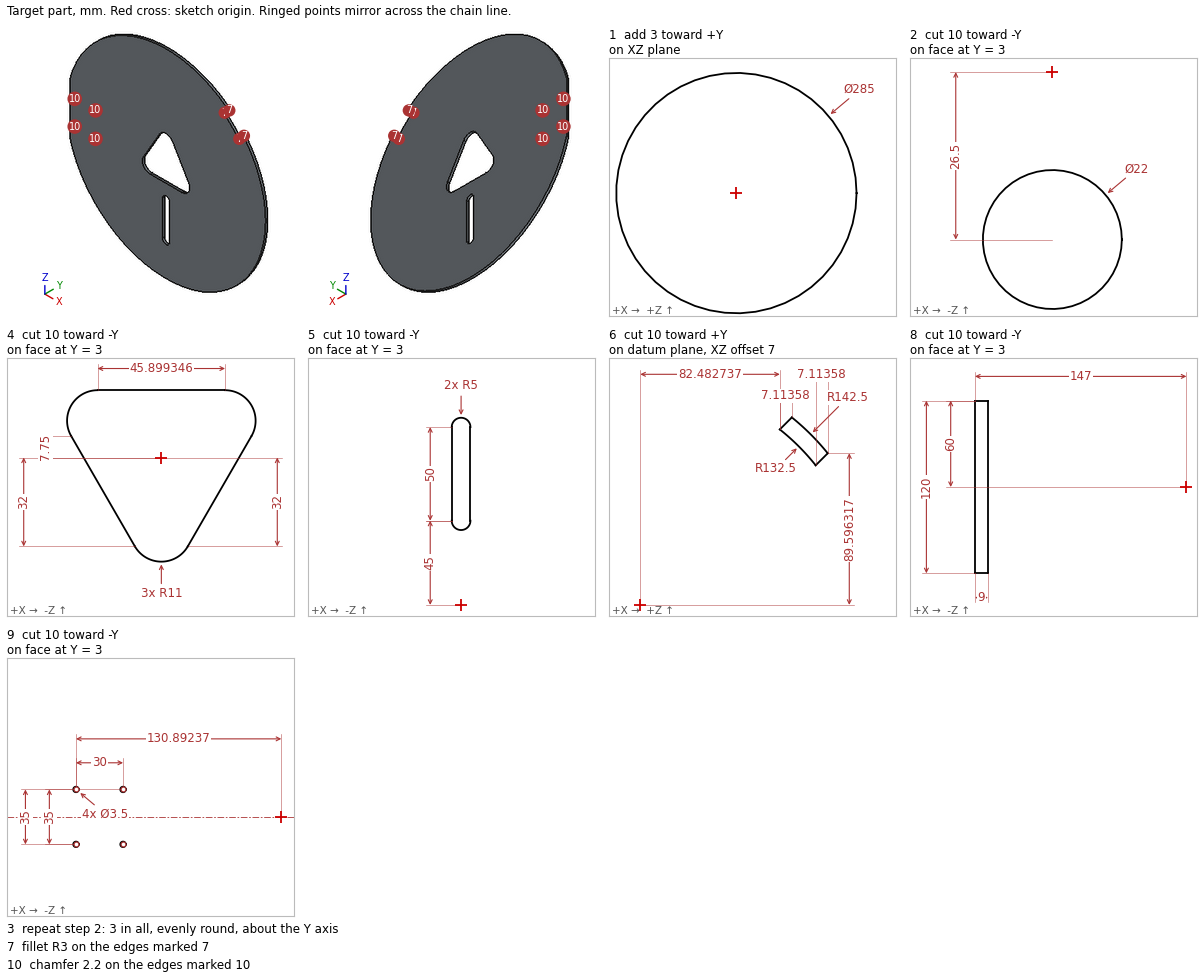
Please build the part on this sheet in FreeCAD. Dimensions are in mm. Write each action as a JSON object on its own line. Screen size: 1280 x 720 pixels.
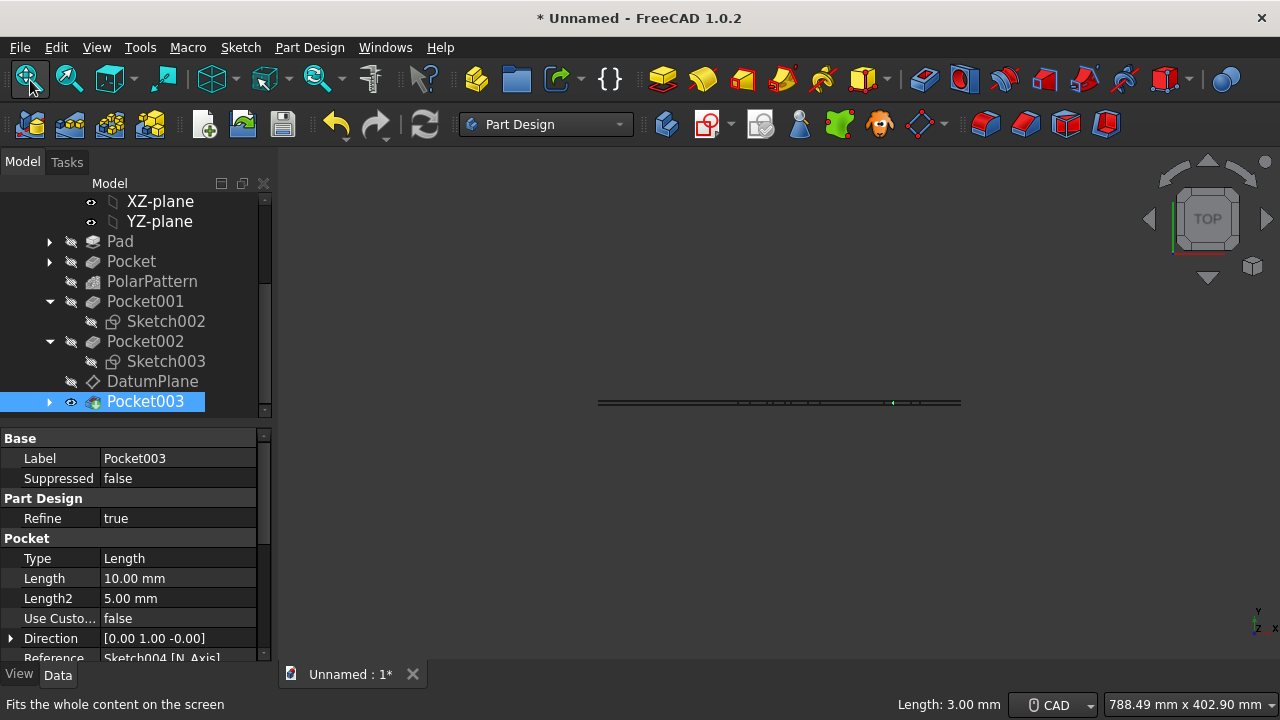
{"action": "scroll", "coordinate": [884, 402], "scroll_direction": "up", "scroll_amount": 12}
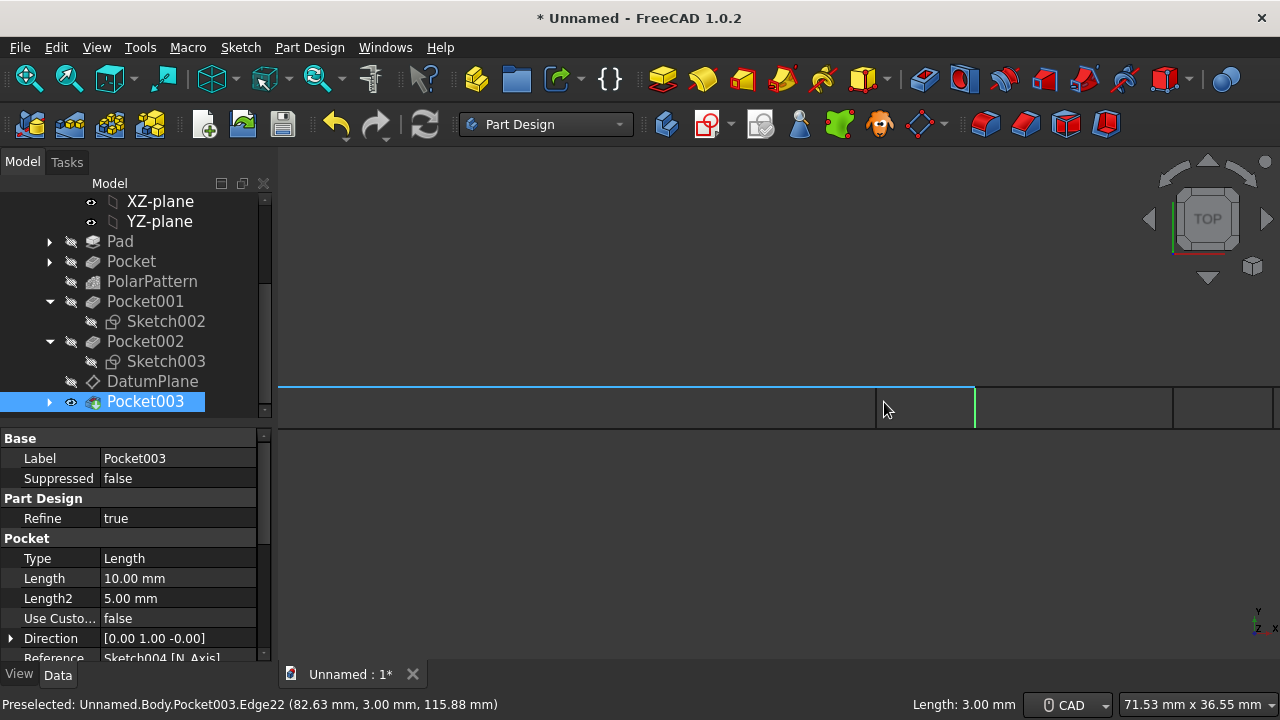
{"action": "left_click", "coordinate": [876, 407], "text": "ctrl"}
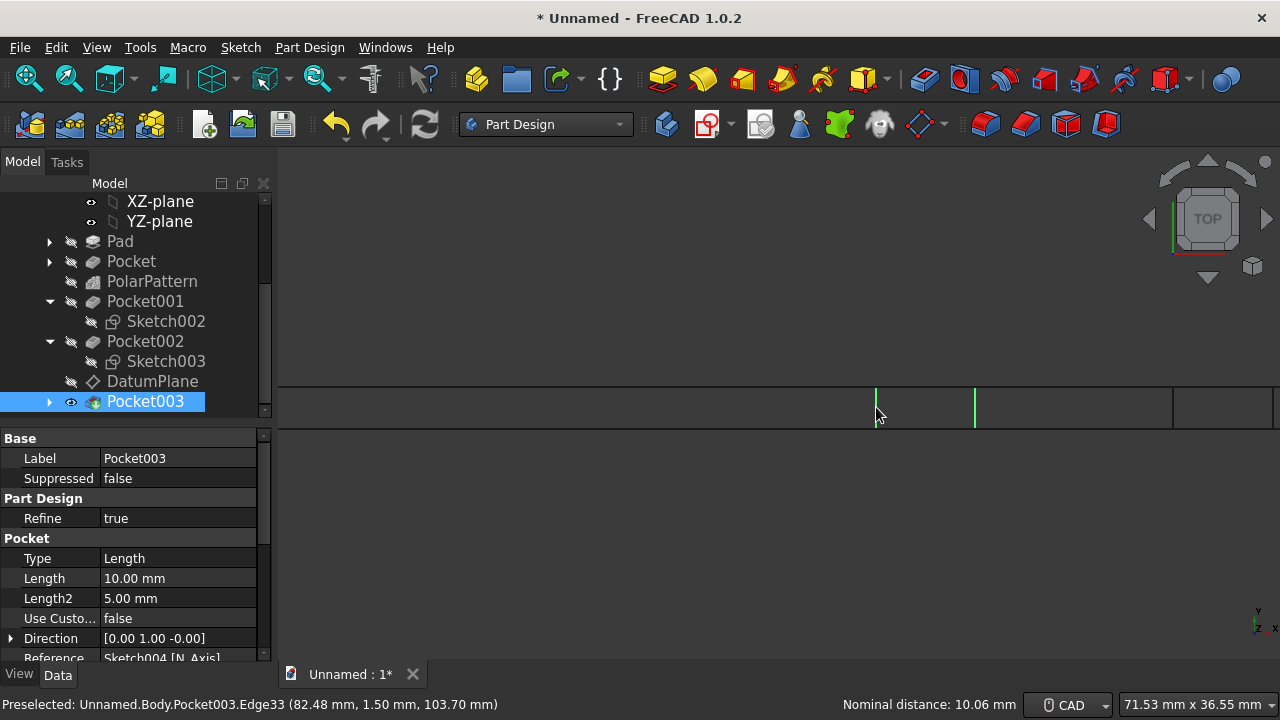
{"action": "left_click", "coordinate": [1173, 407], "text": "ctrl"}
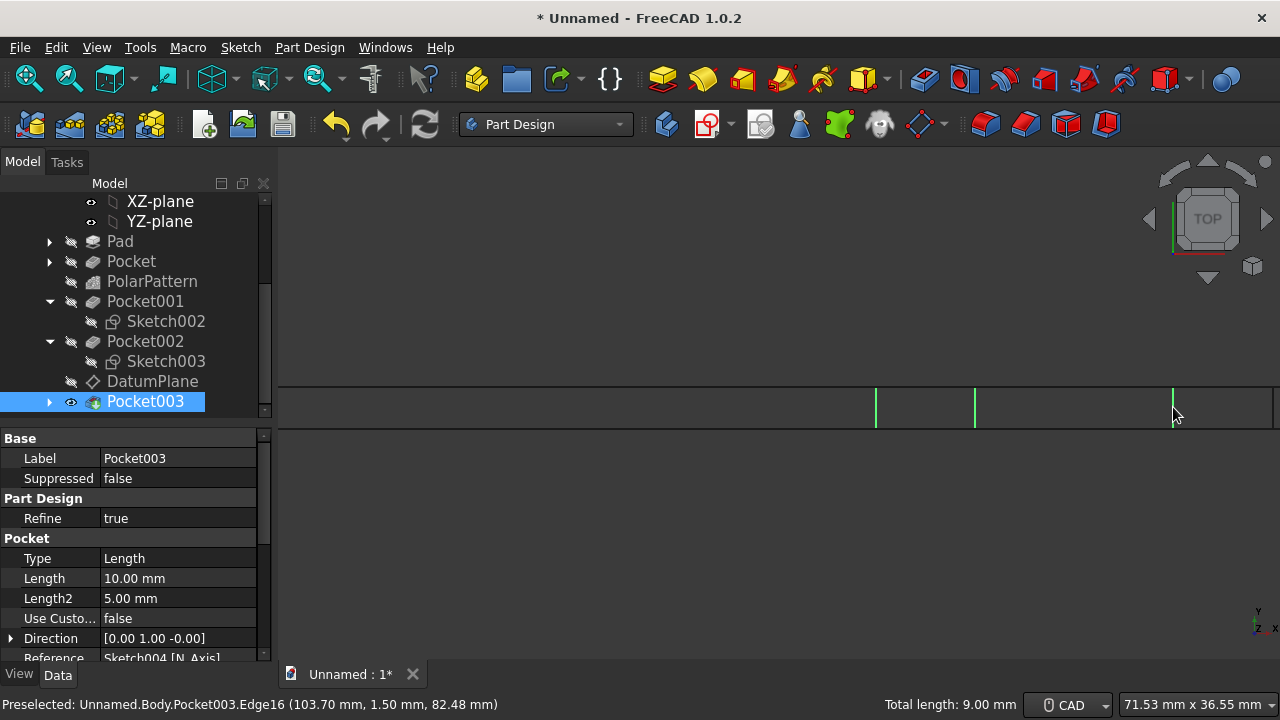
{"action": "left_click", "coordinate": [30, 80]}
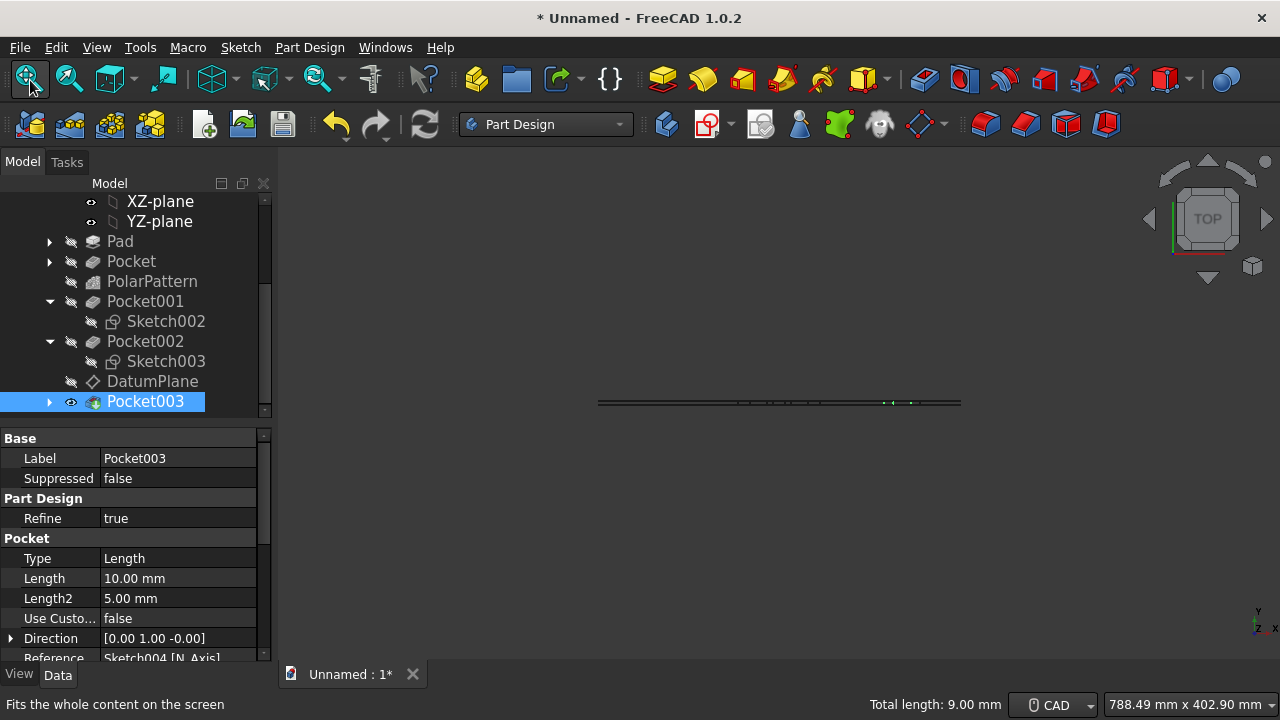
{"action": "key", "text": "1"}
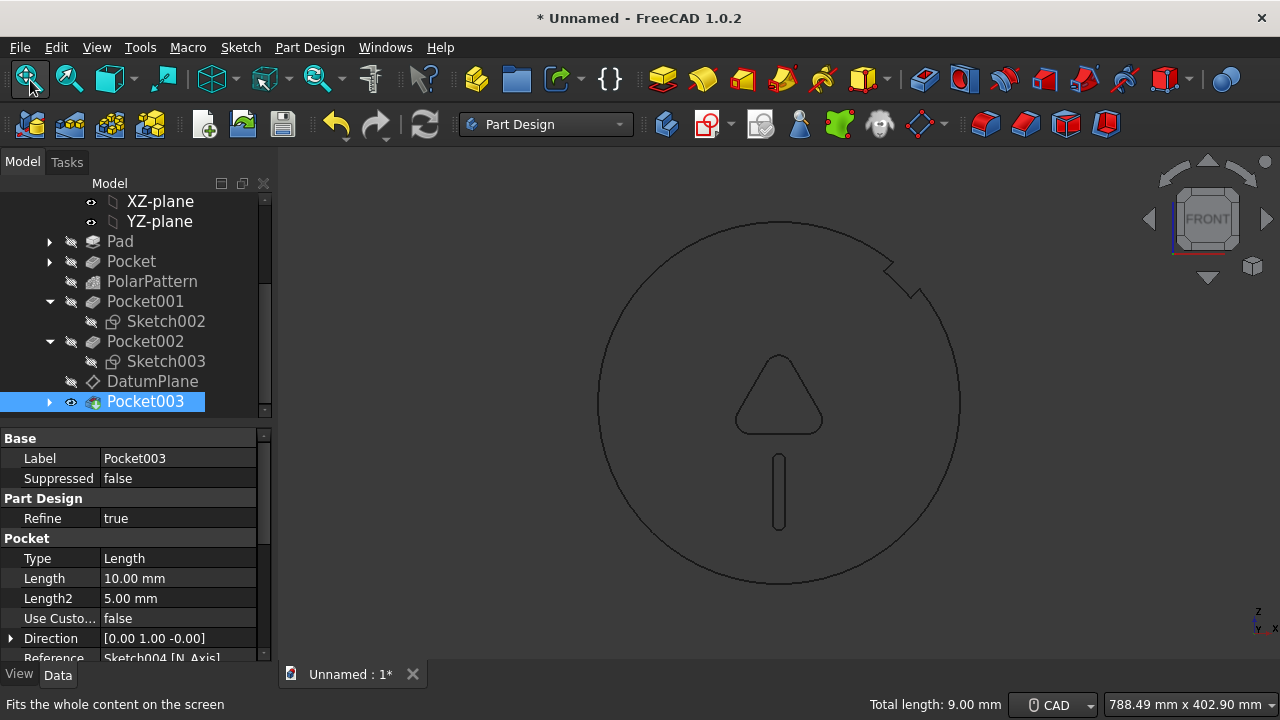
{"action": "scroll", "coordinate": [920, 288], "scroll_direction": "up", "scroll_amount": 12}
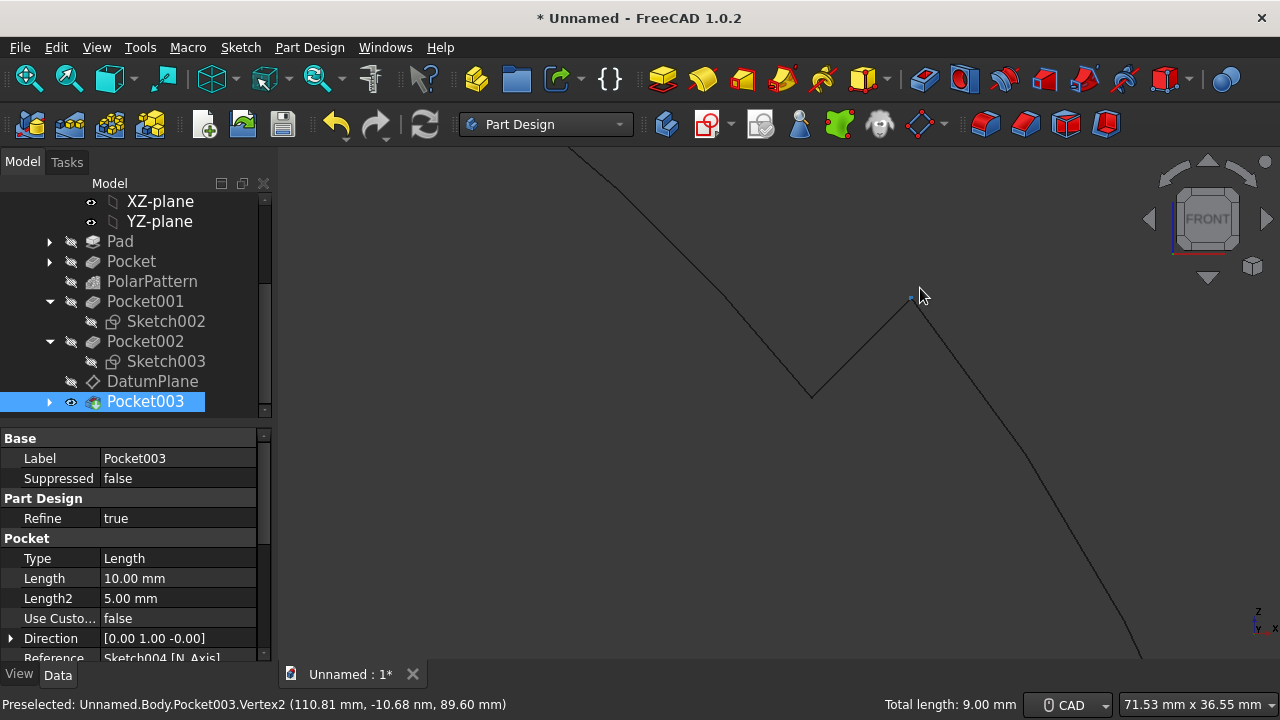
{"action": "left_click", "coordinate": [30, 80]}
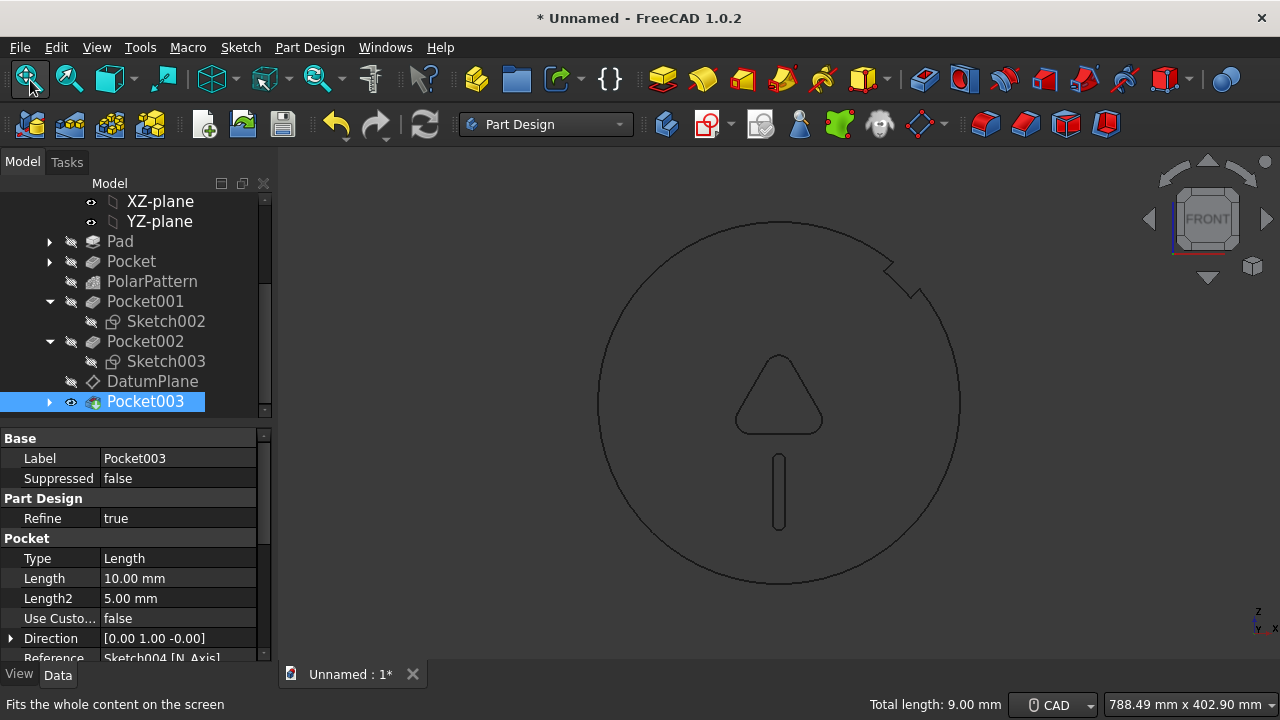
{"action": "key", "text": "3"}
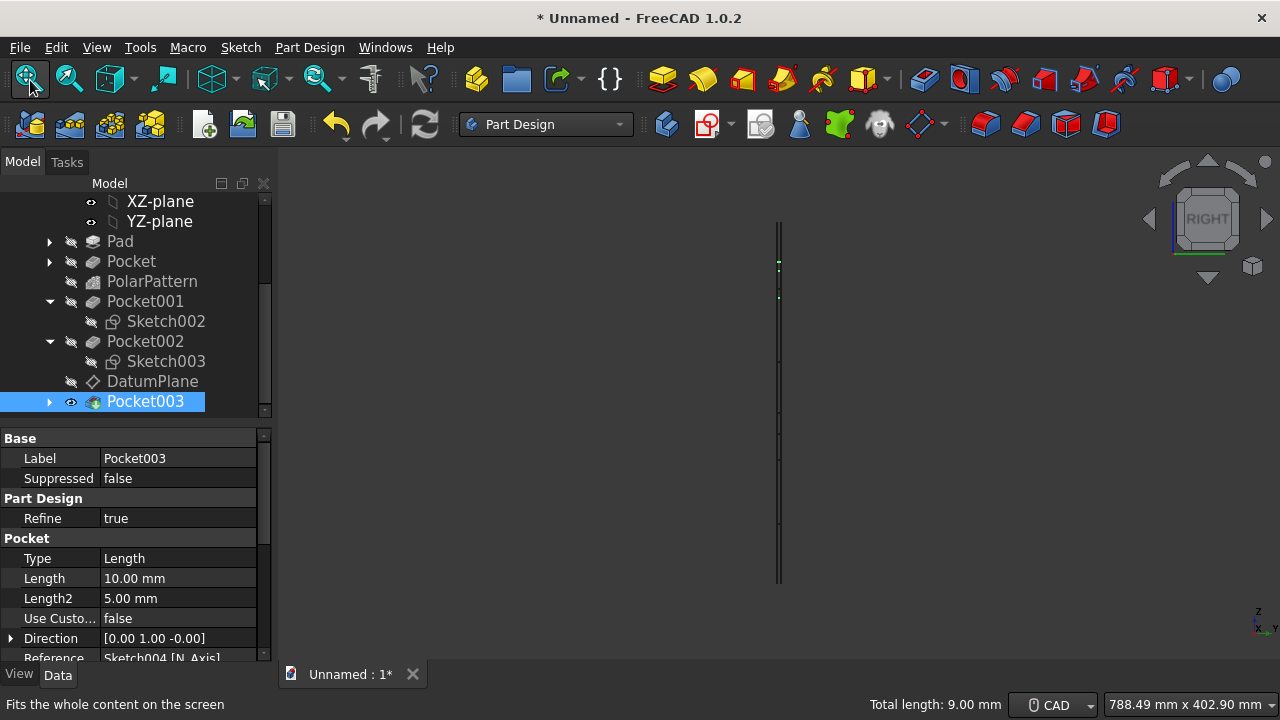
{"action": "scroll", "coordinate": [779, 288], "scroll_direction": "up", "scroll_amount": 12}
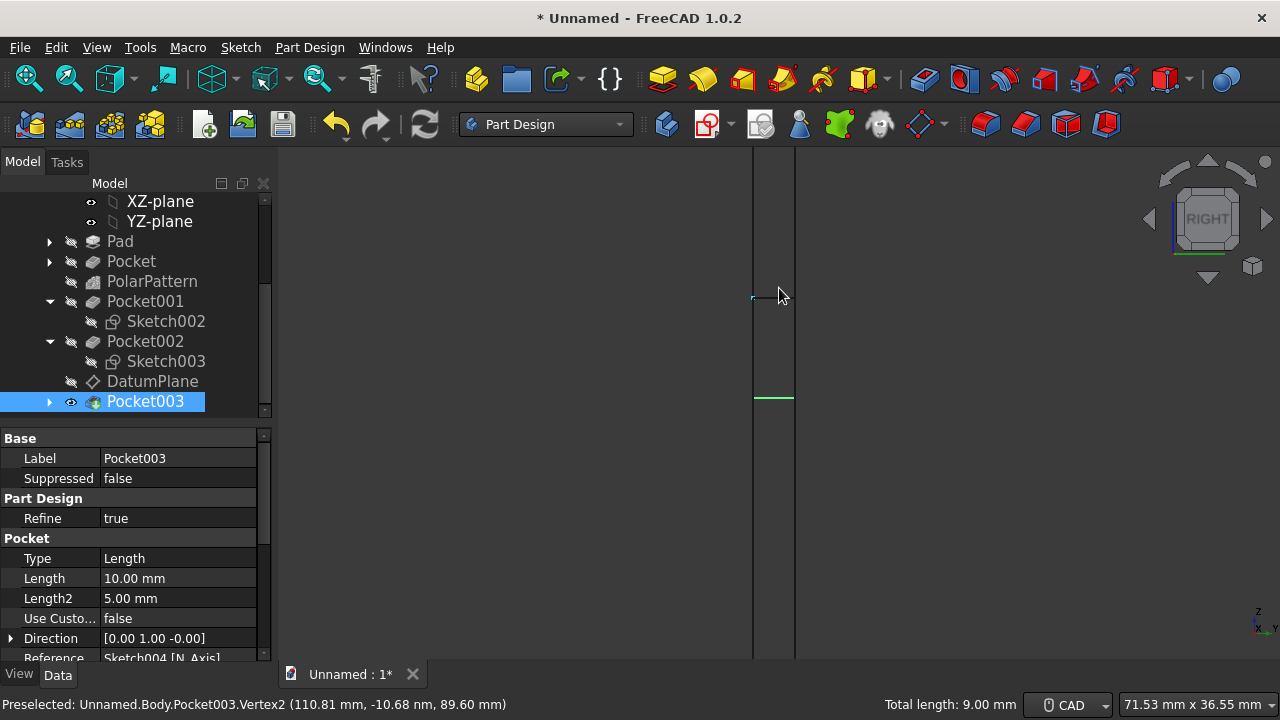
{"action": "left_click", "coordinate": [774, 297], "text": "ctrl"}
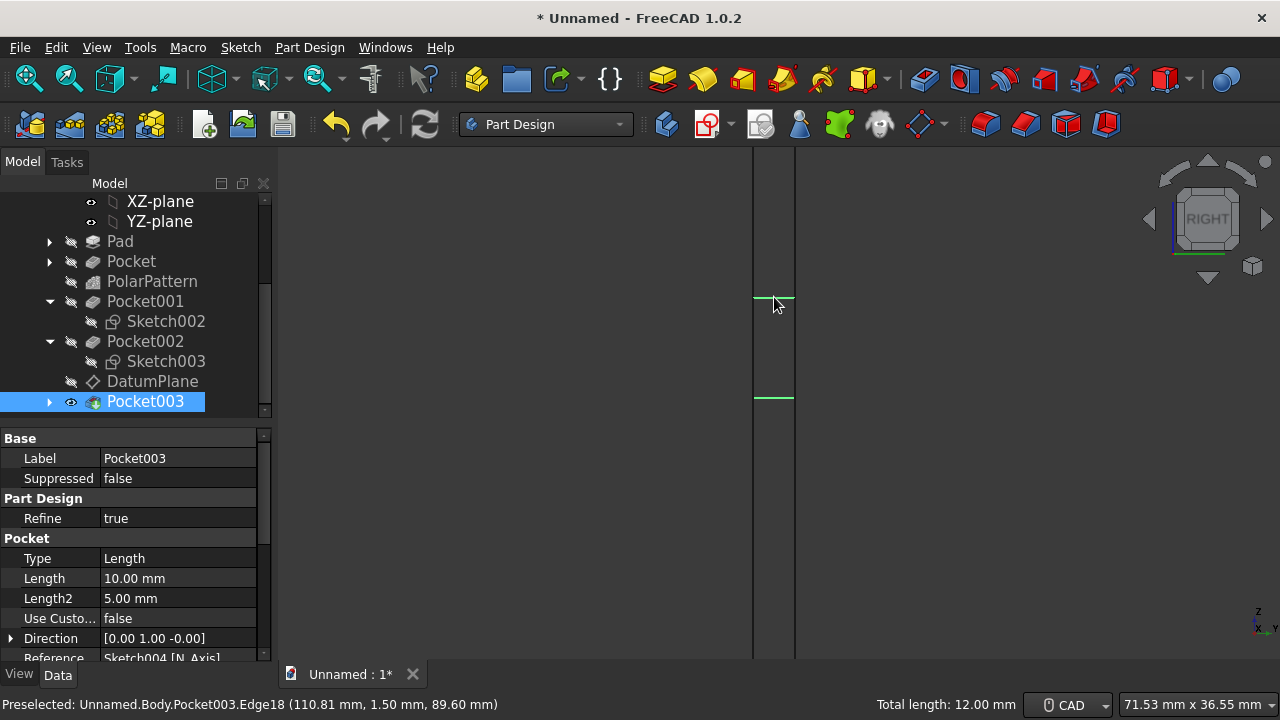
{"action": "key", "text": "v 1"}